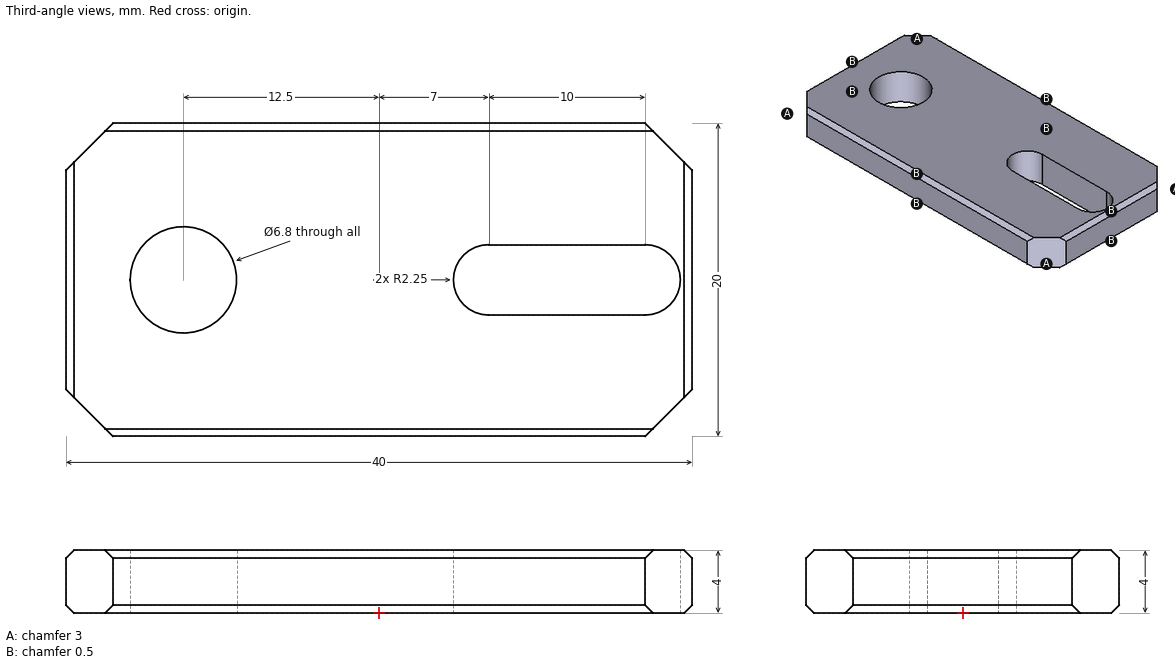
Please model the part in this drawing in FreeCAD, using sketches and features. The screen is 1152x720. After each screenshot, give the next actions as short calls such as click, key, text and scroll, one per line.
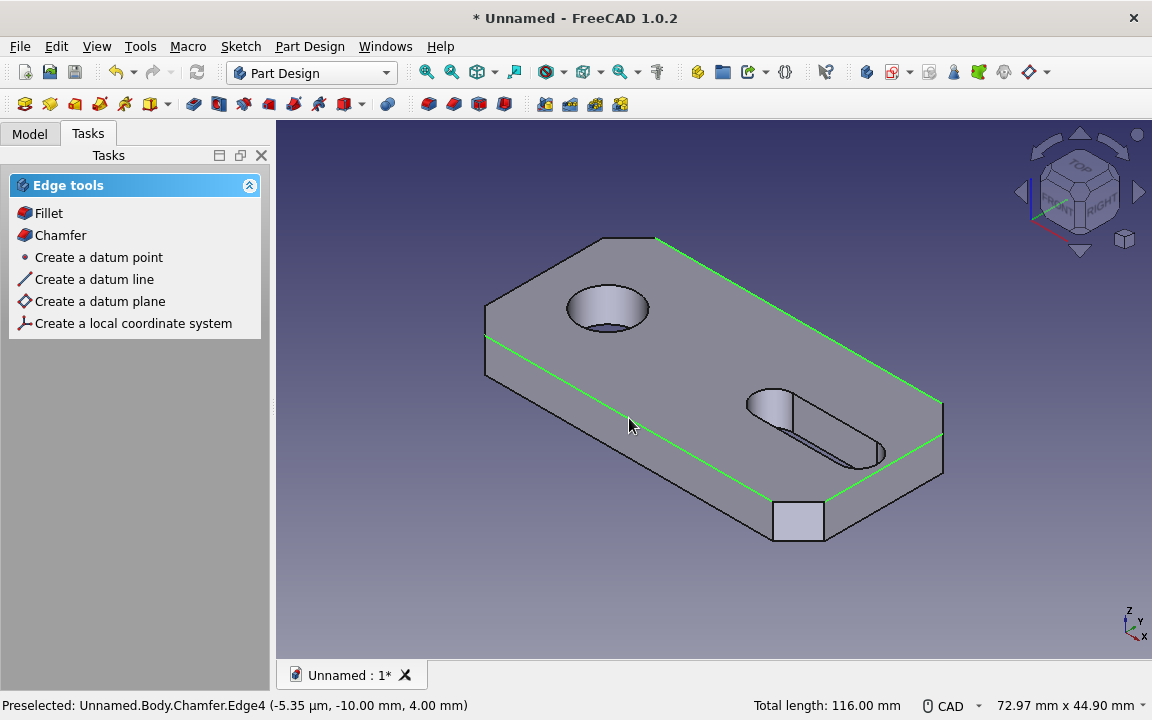
key(2)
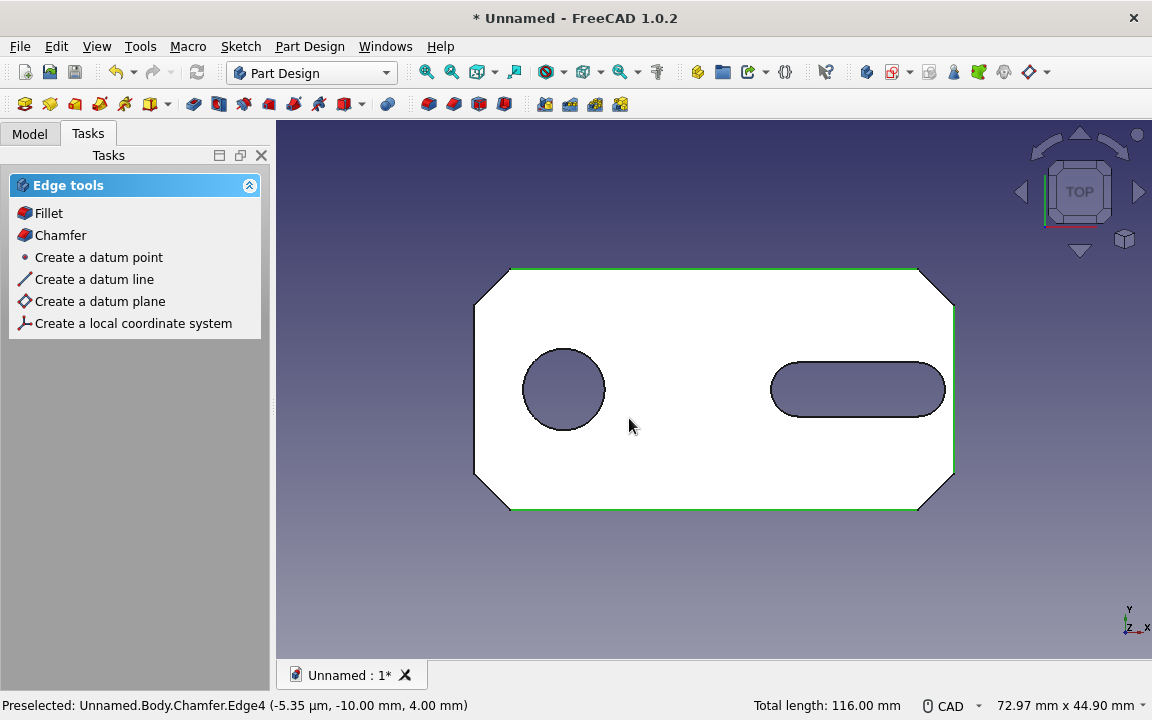
click(474, 389, ctrl)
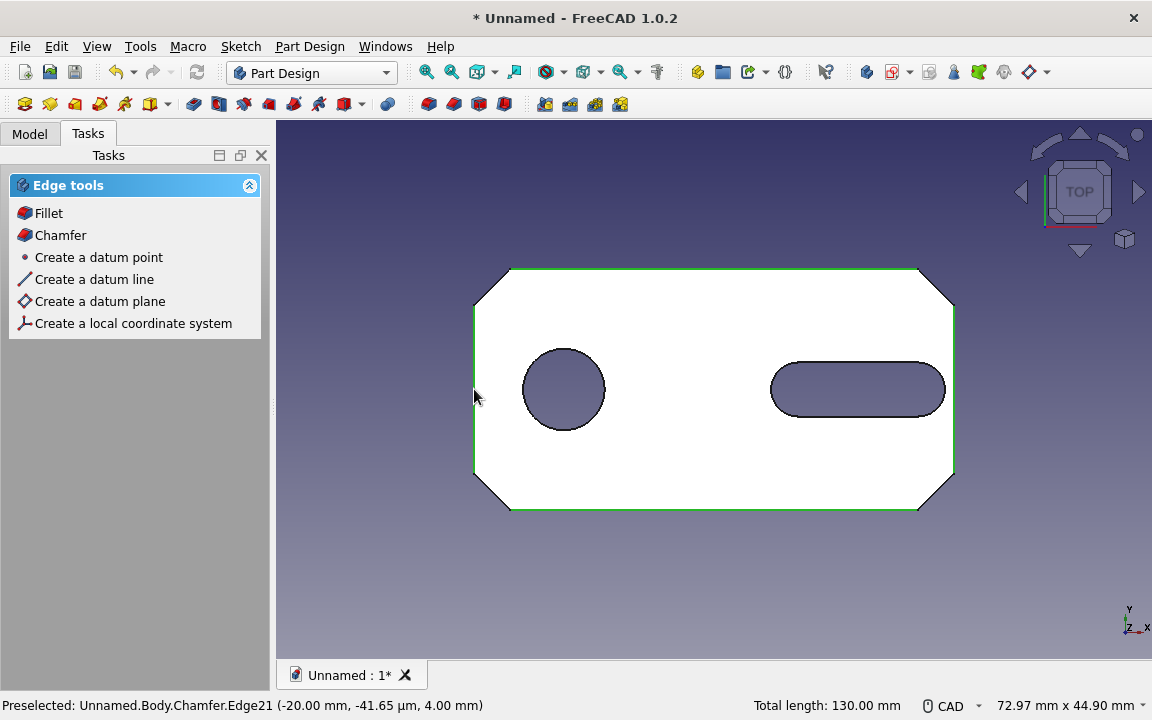
key(1)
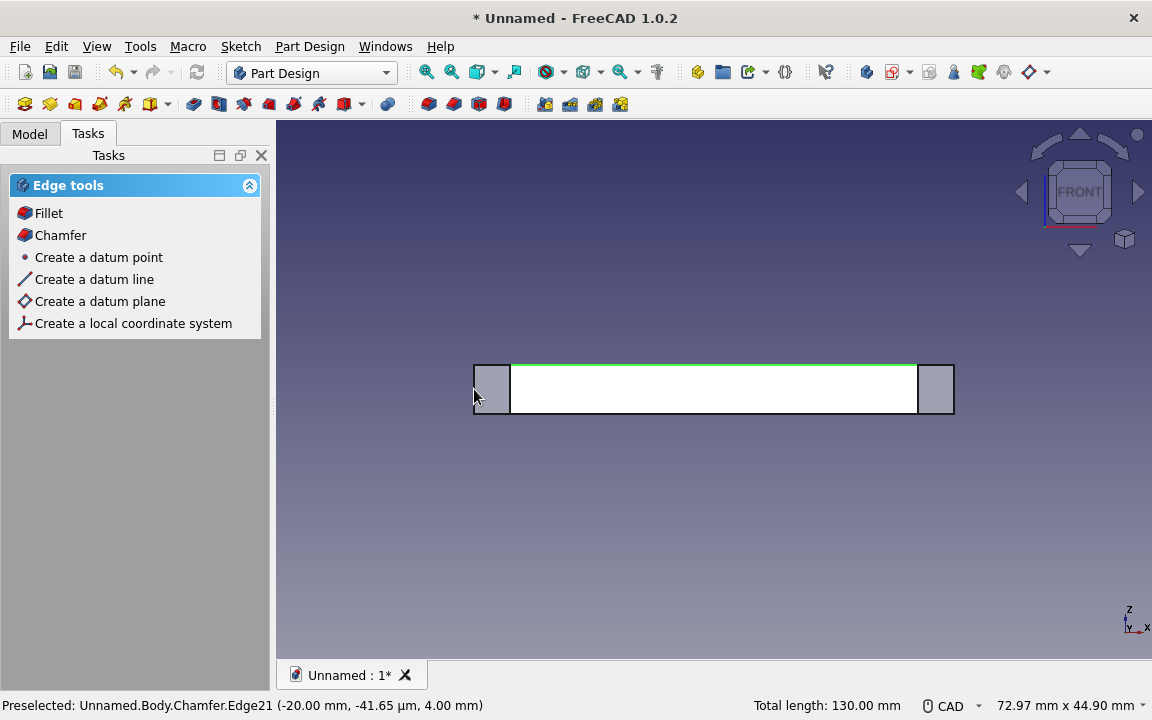
click(714, 413, ctrl)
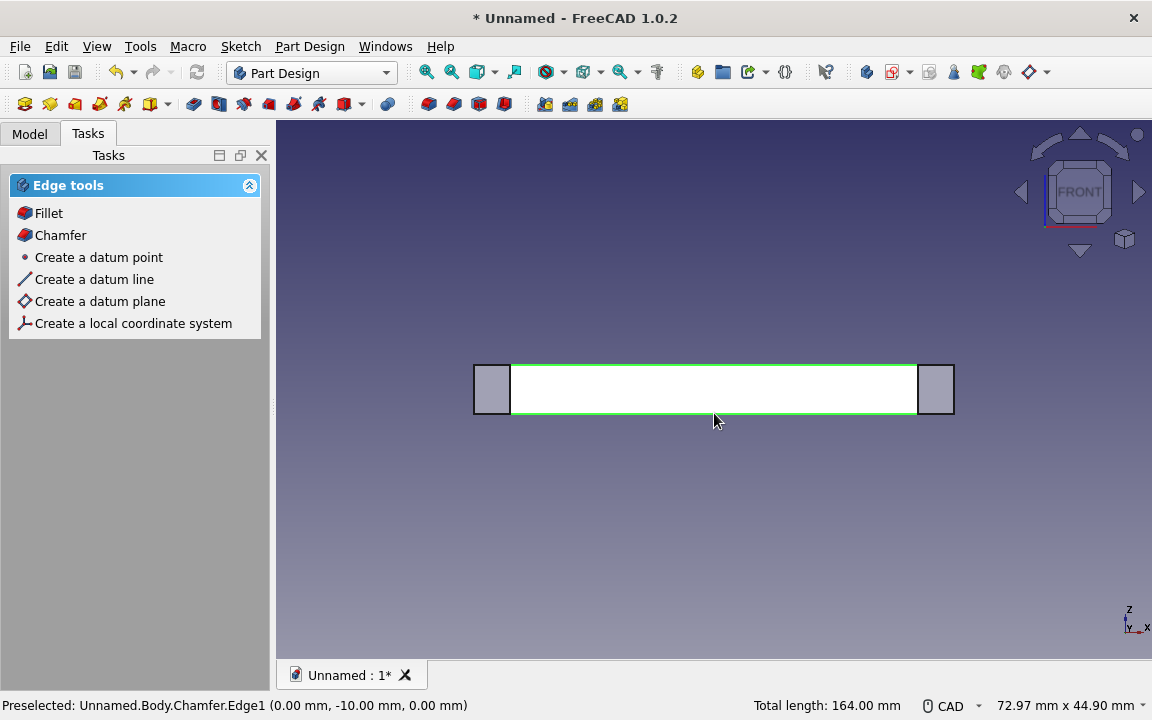
key(3)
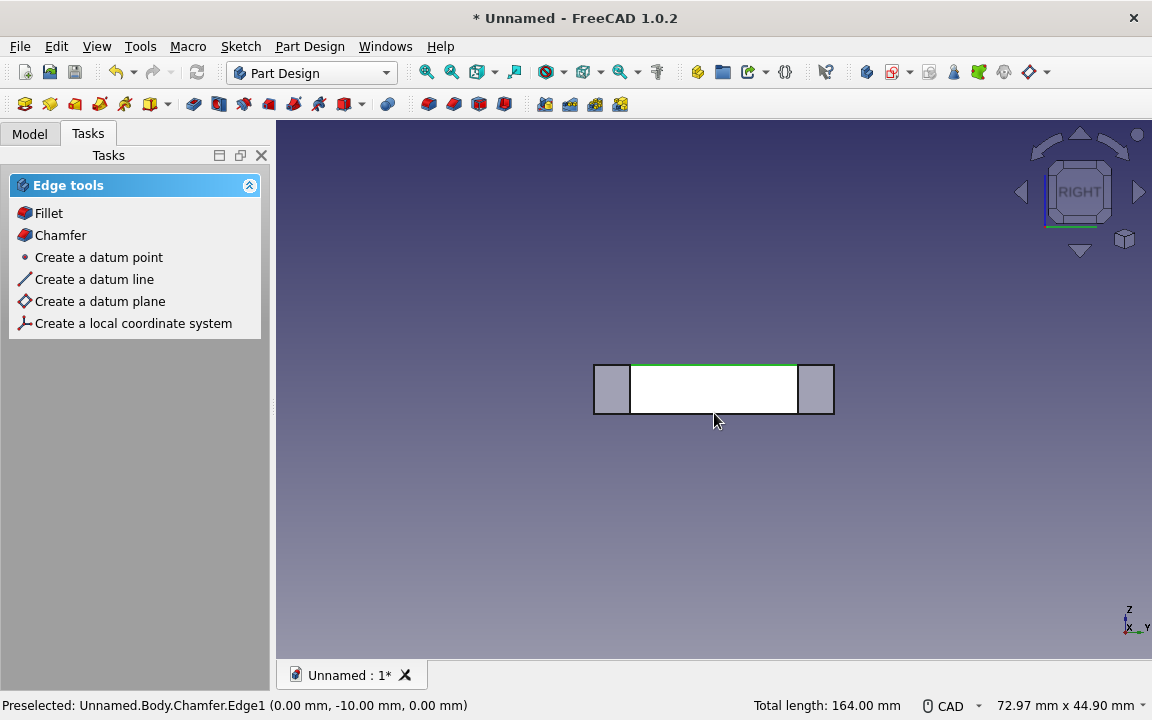
click(427, 72)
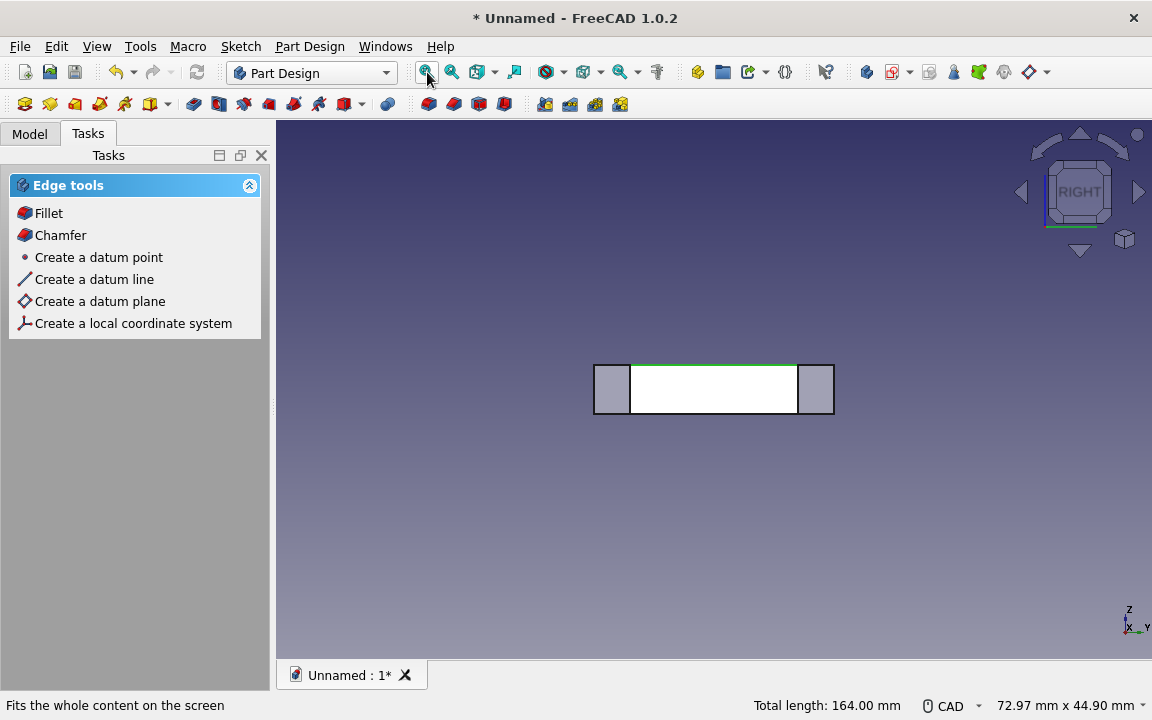
click(714, 413, ctrl)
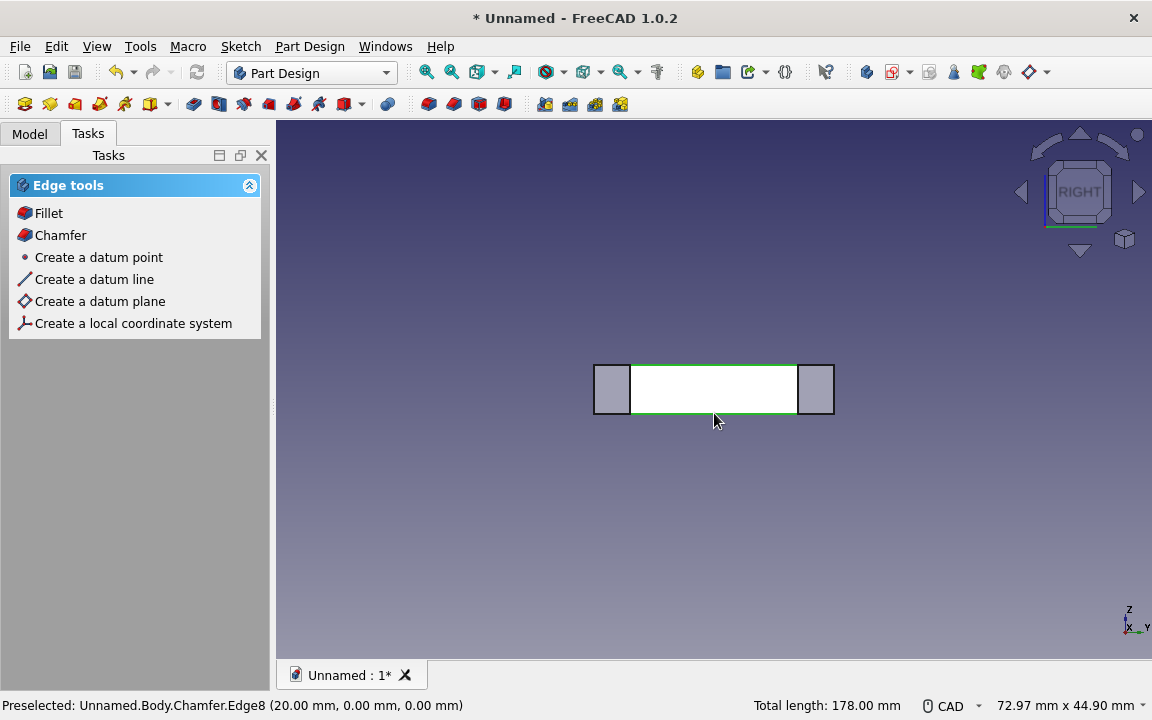
key(5)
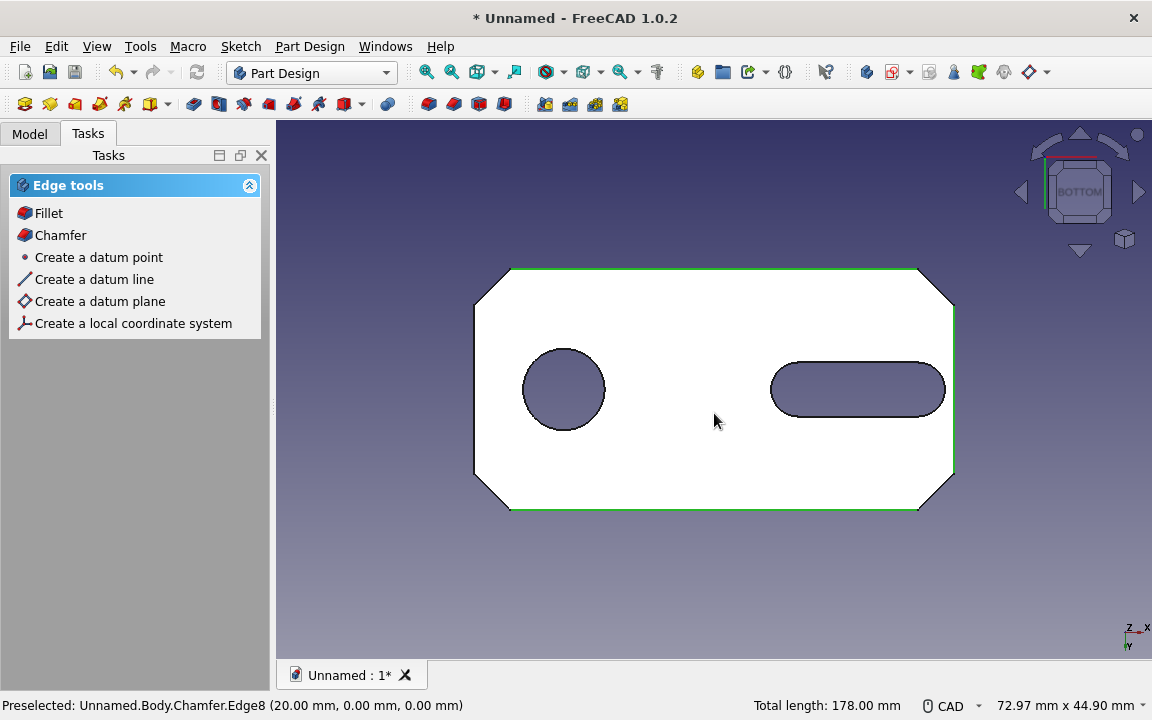
click(474, 388, ctrl)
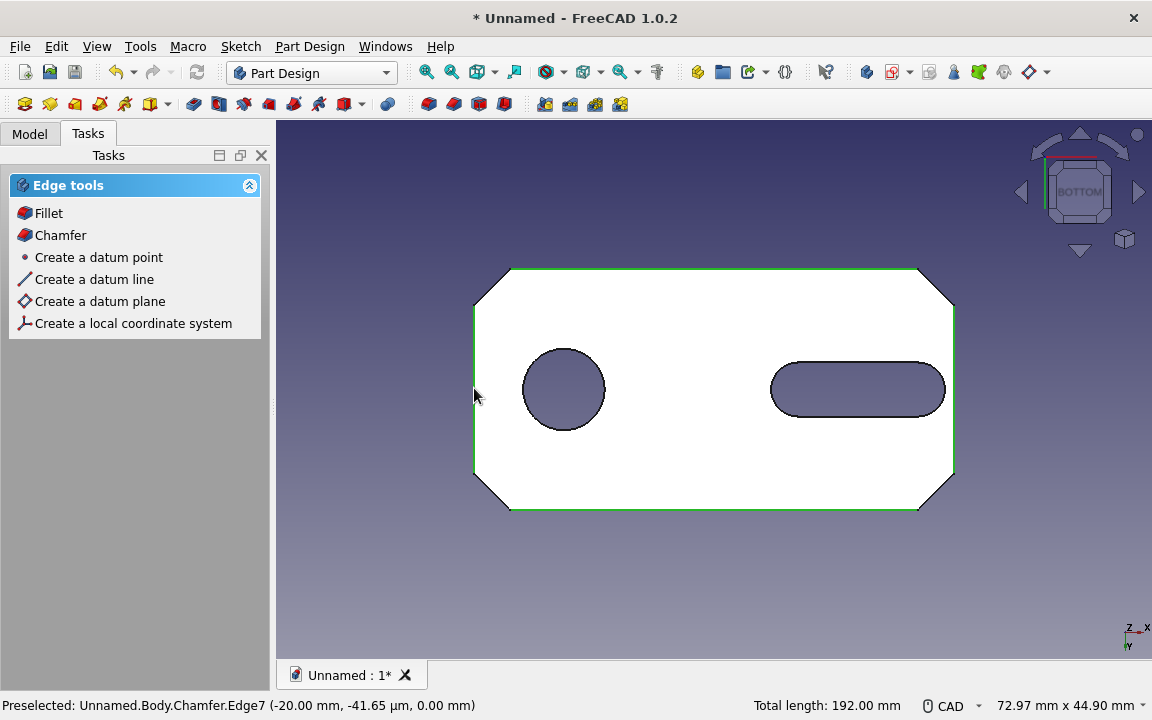
click(454, 104)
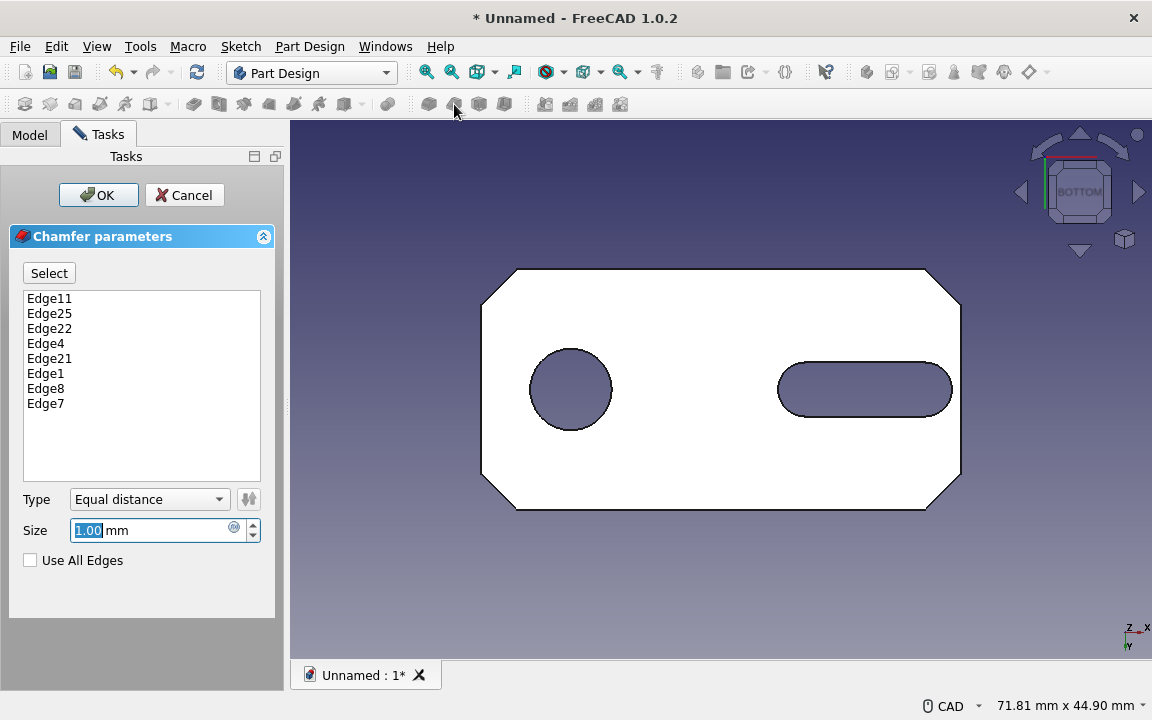
text(0.5)
key(Tab)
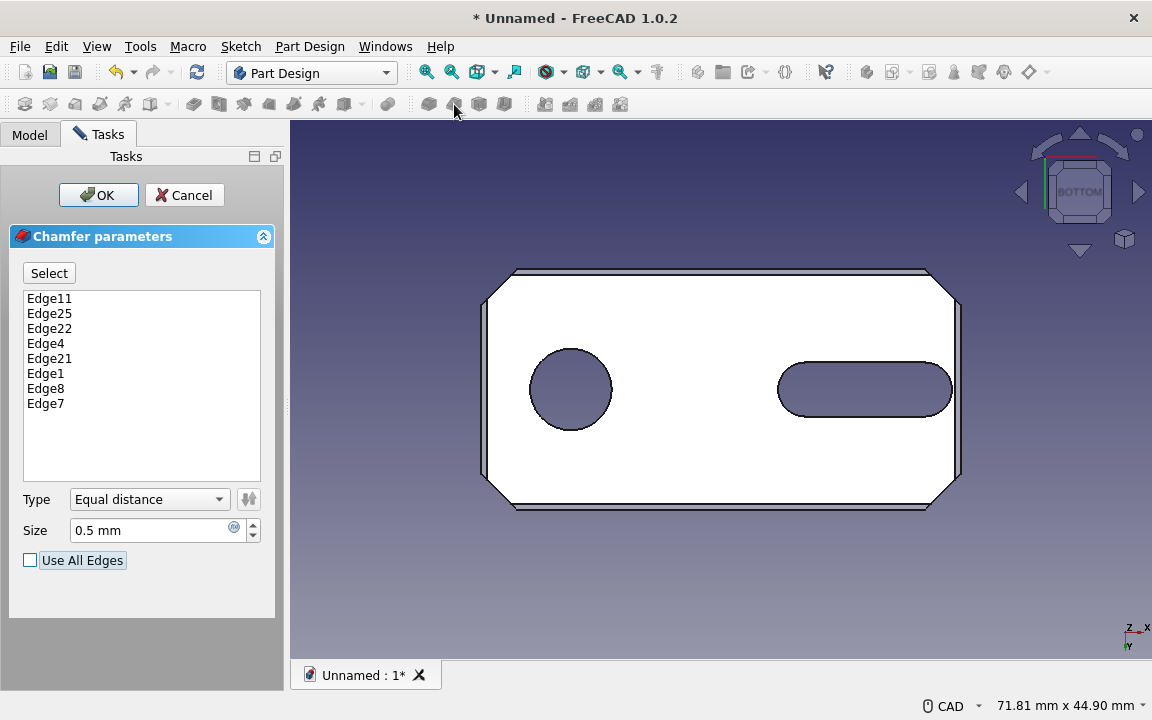
click(99, 195)